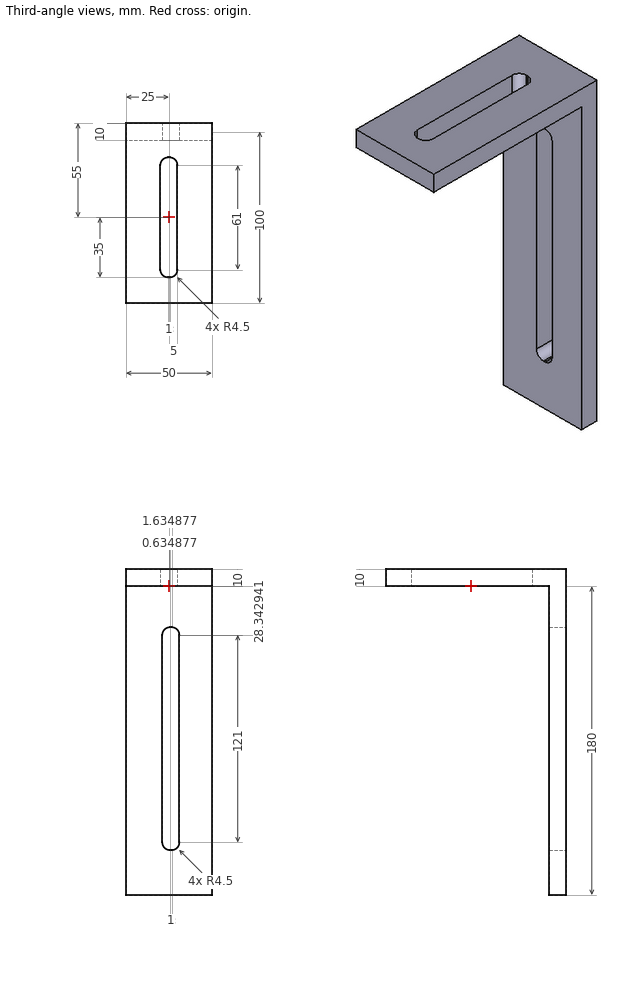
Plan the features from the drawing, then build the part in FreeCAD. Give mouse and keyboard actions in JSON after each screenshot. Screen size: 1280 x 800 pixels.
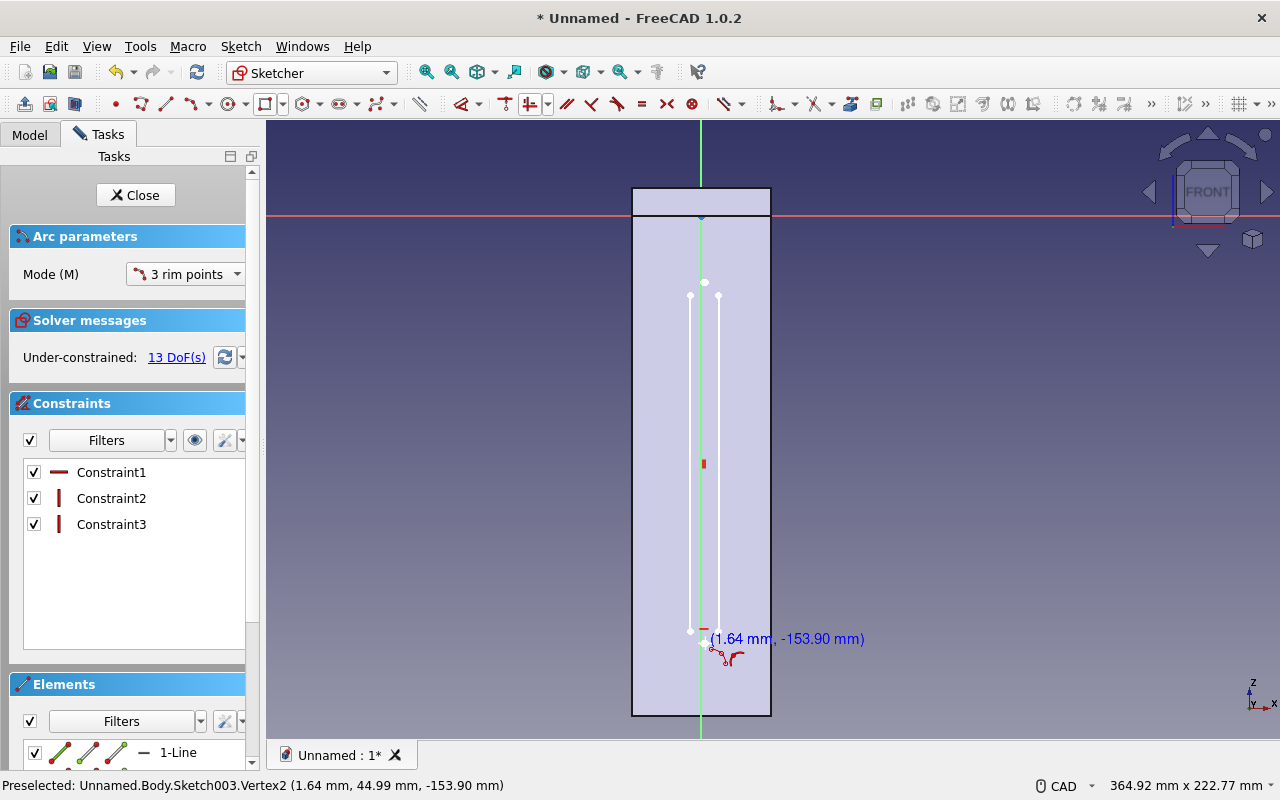
{"action": "left_click", "coordinate": [719, 632]}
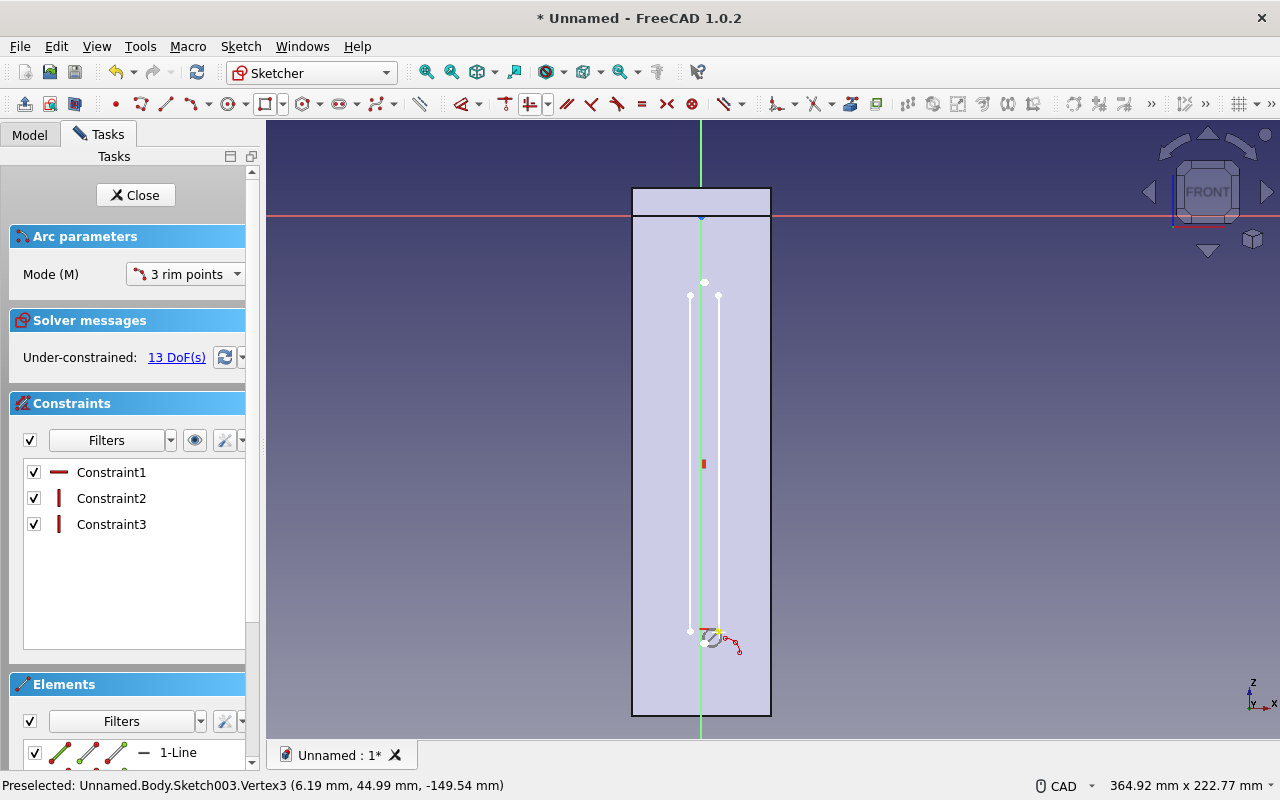
{"action": "scroll", "coordinate": [715, 640], "scroll_direction": "up", "scroll_amount": 8}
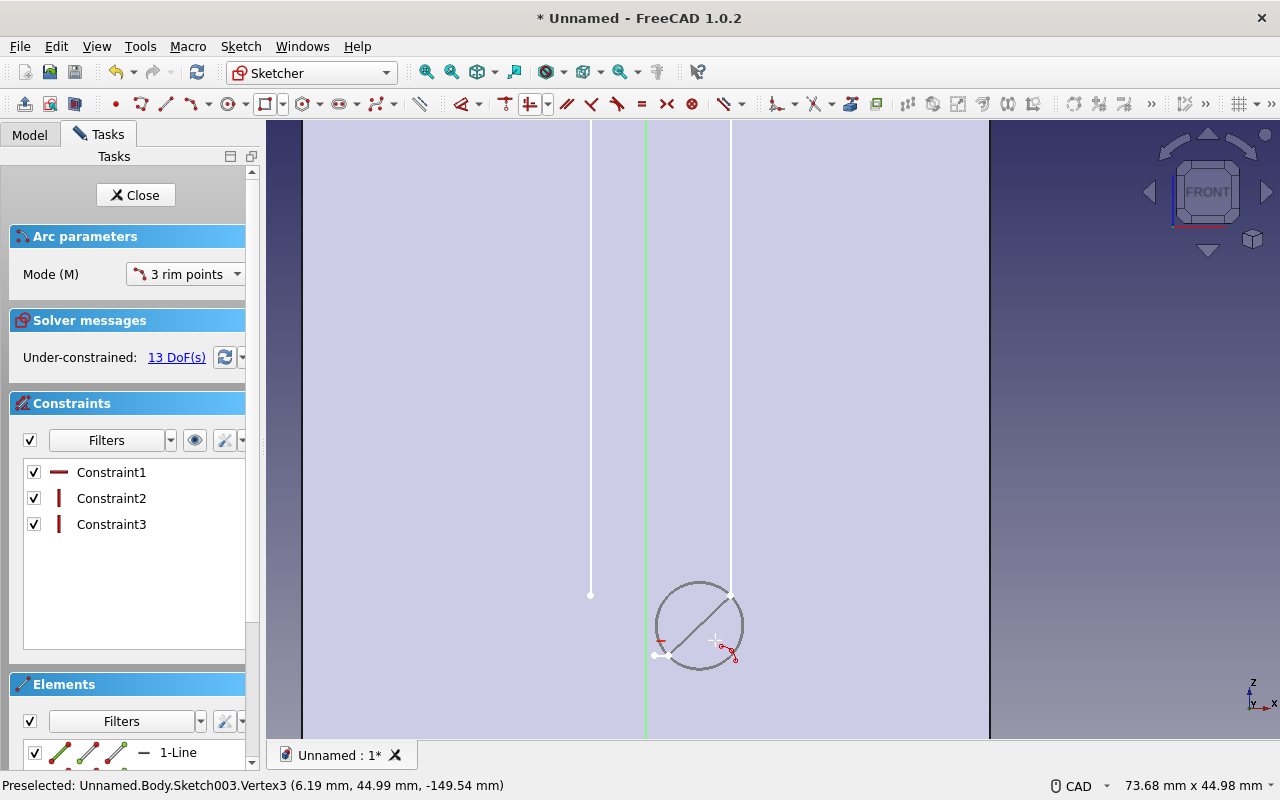
{"action": "left_click", "coordinate": [712, 637]}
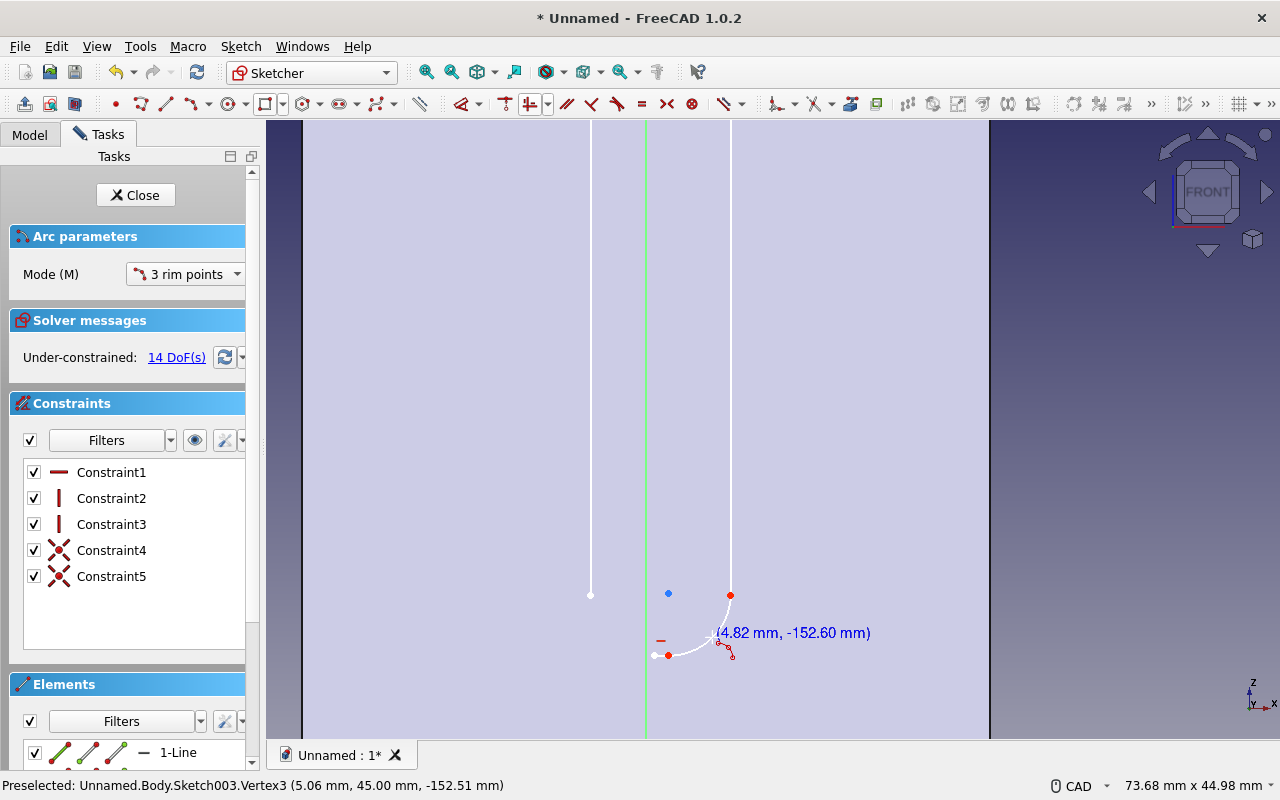
{"action": "scroll", "coordinate": [715, 640], "scroll_direction": "down", "scroll_amount": 8}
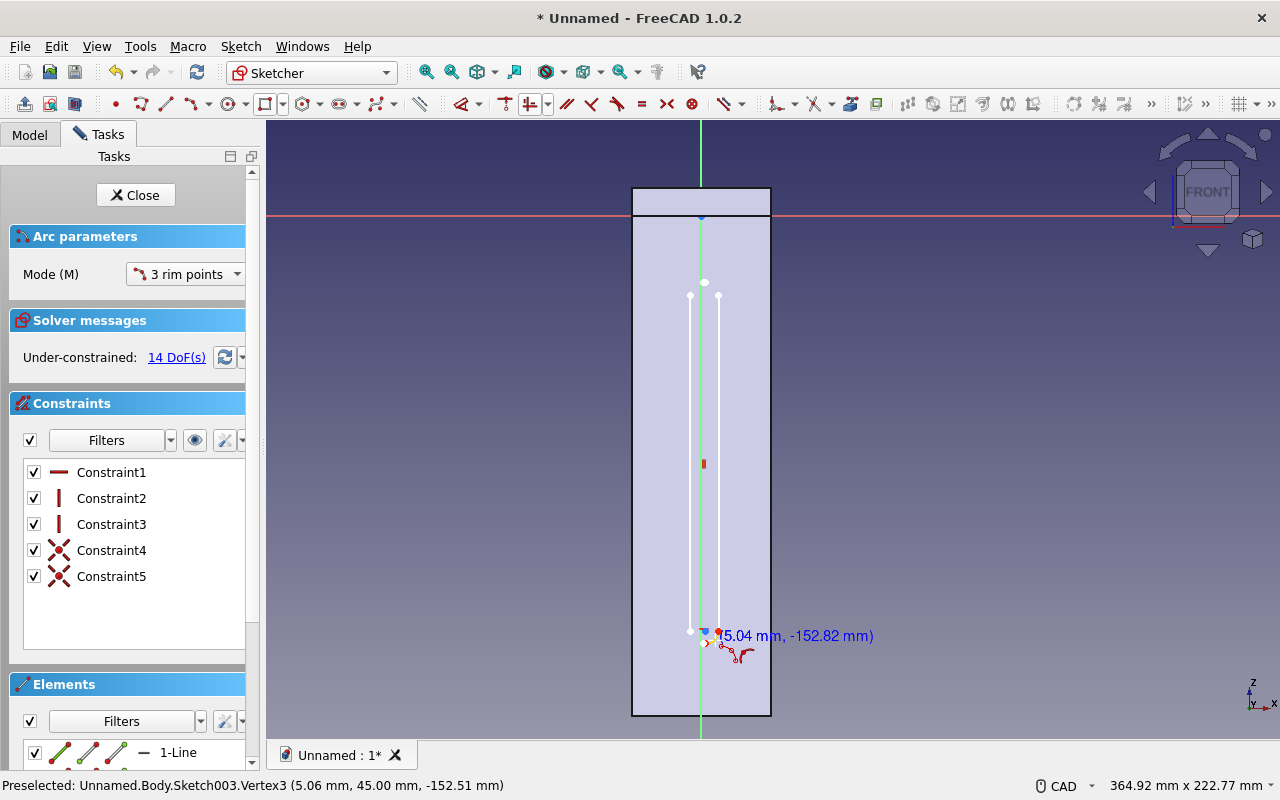
{"action": "left_click", "coordinate": [719, 296]}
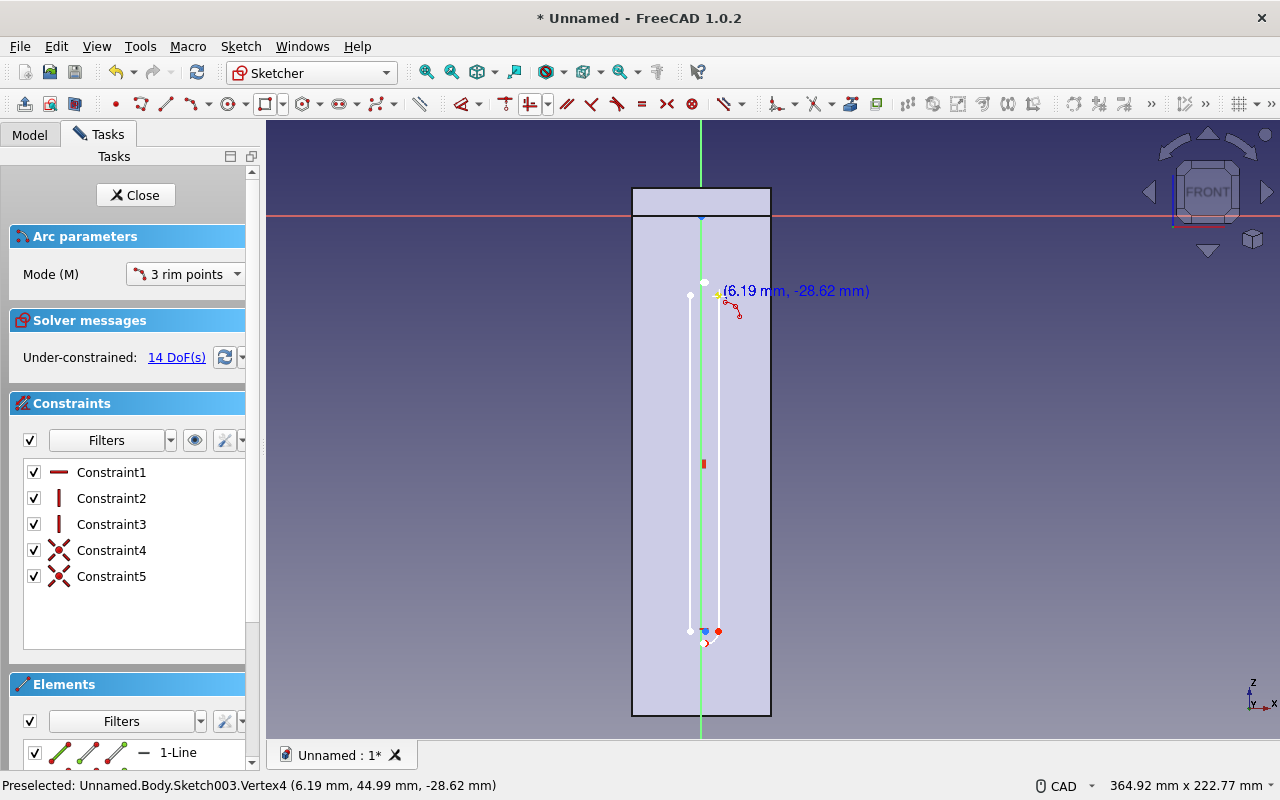
{"action": "scroll", "coordinate": [706, 282], "scroll_direction": "up", "scroll_amount": 13}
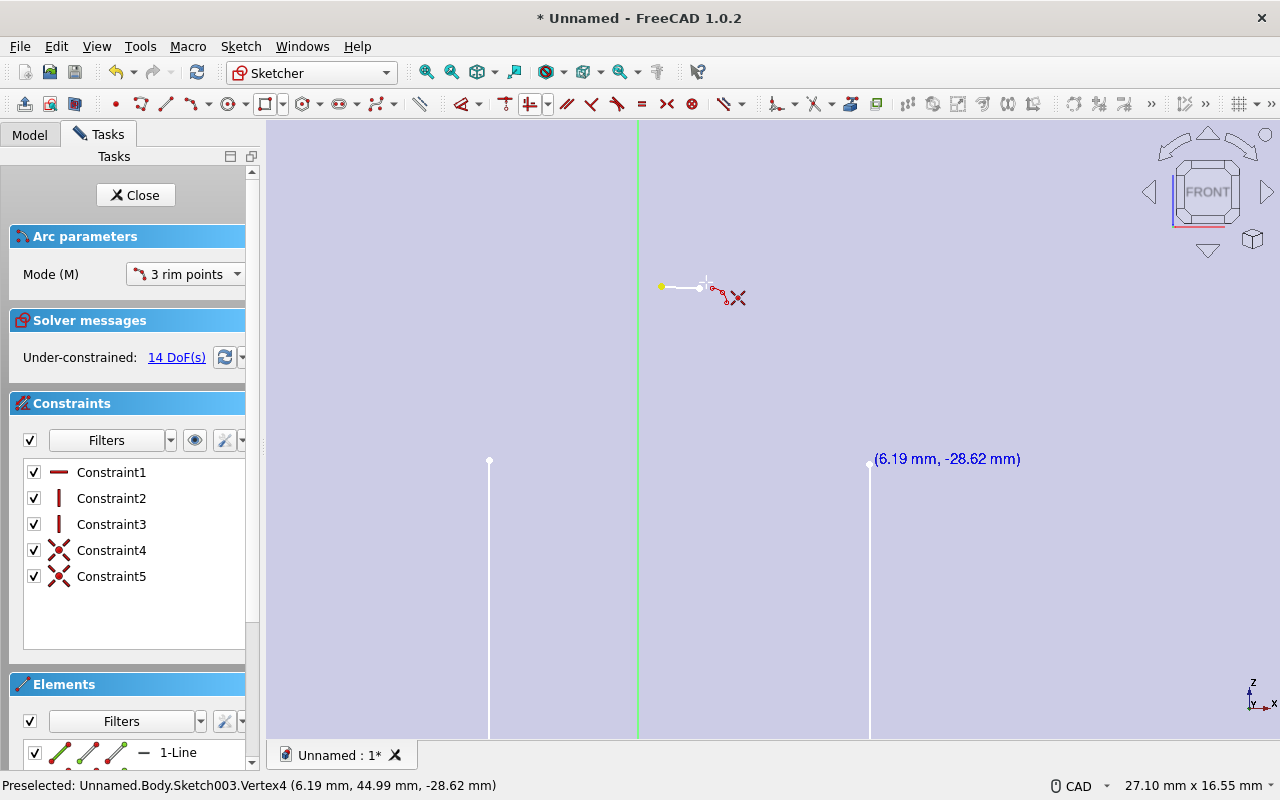
{"action": "left_click", "coordinate": [699, 288]}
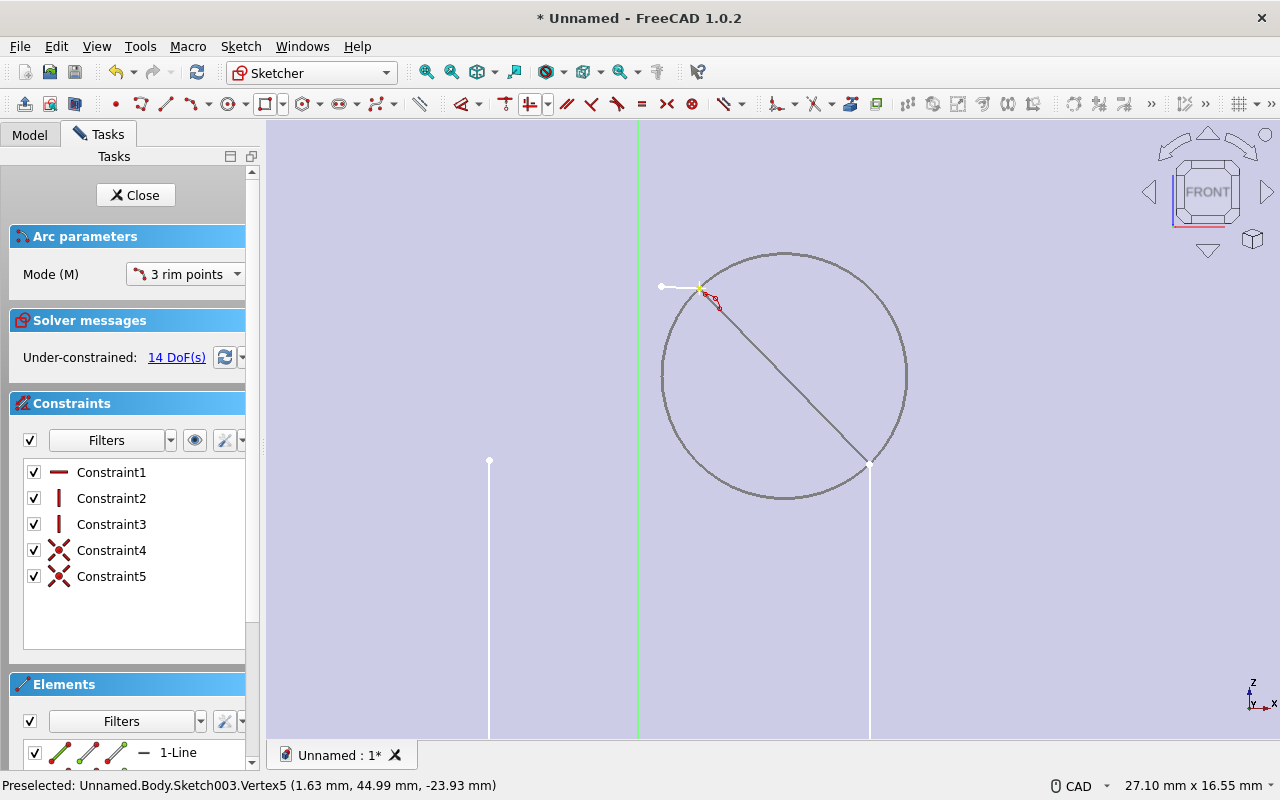
{"action": "scroll", "coordinate": [706, 282], "scroll_direction": "down", "scroll_amount": 13}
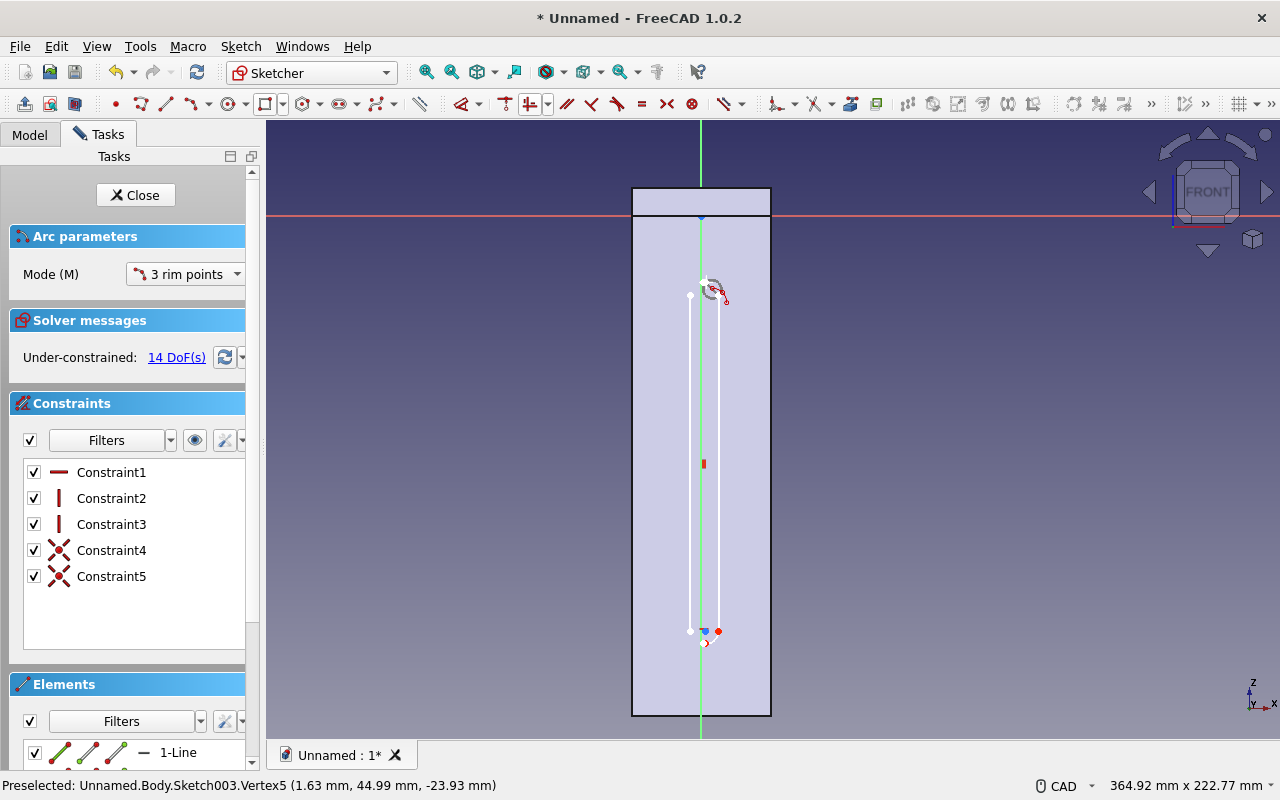
{"action": "scroll", "coordinate": [715, 286], "scroll_direction": "up", "scroll_amount": 8}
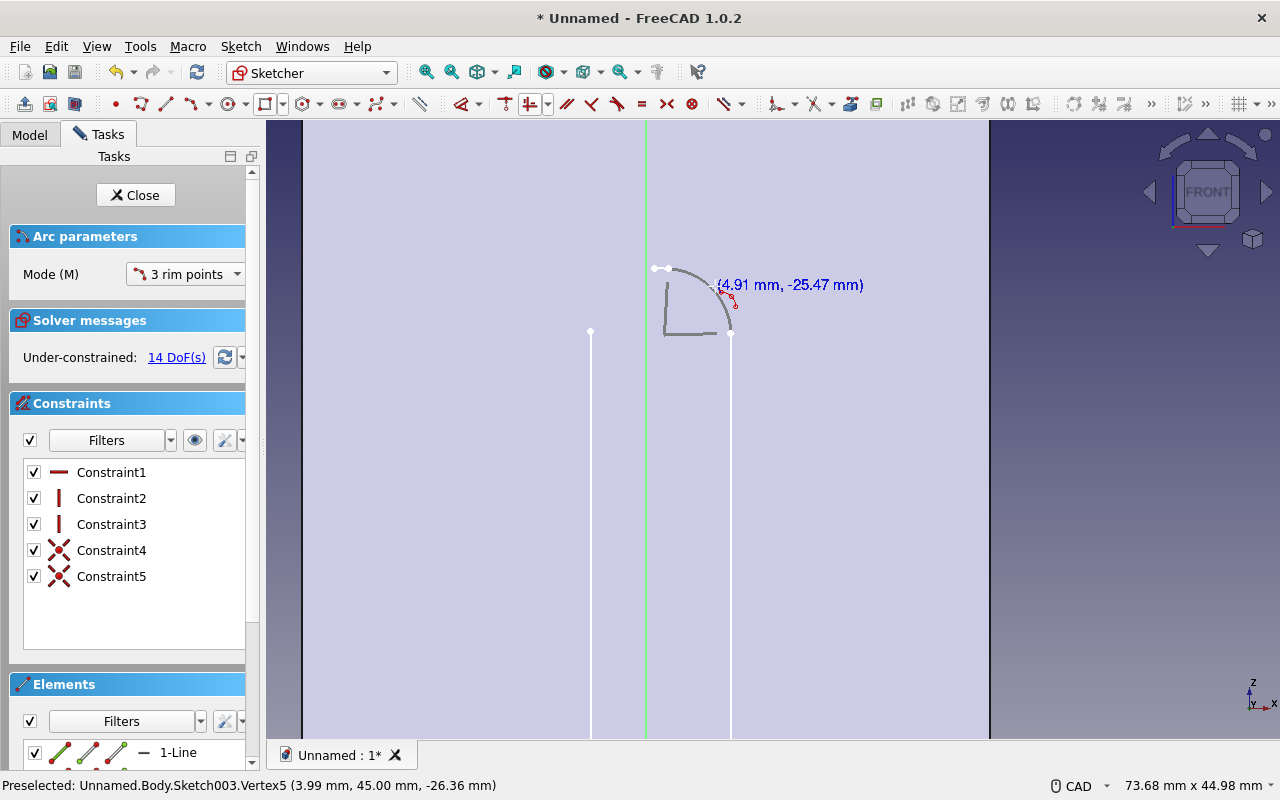
{"action": "left_click", "coordinate": [712, 286]}